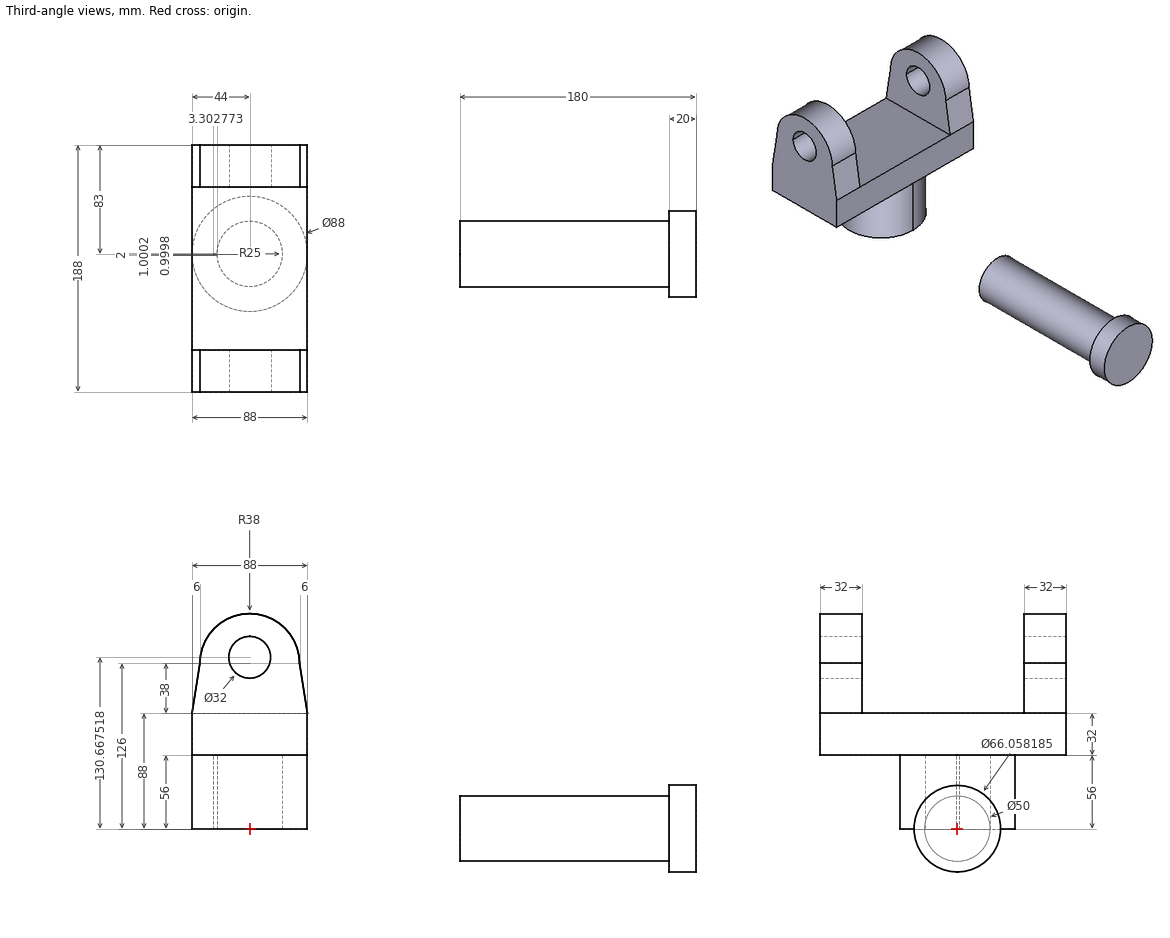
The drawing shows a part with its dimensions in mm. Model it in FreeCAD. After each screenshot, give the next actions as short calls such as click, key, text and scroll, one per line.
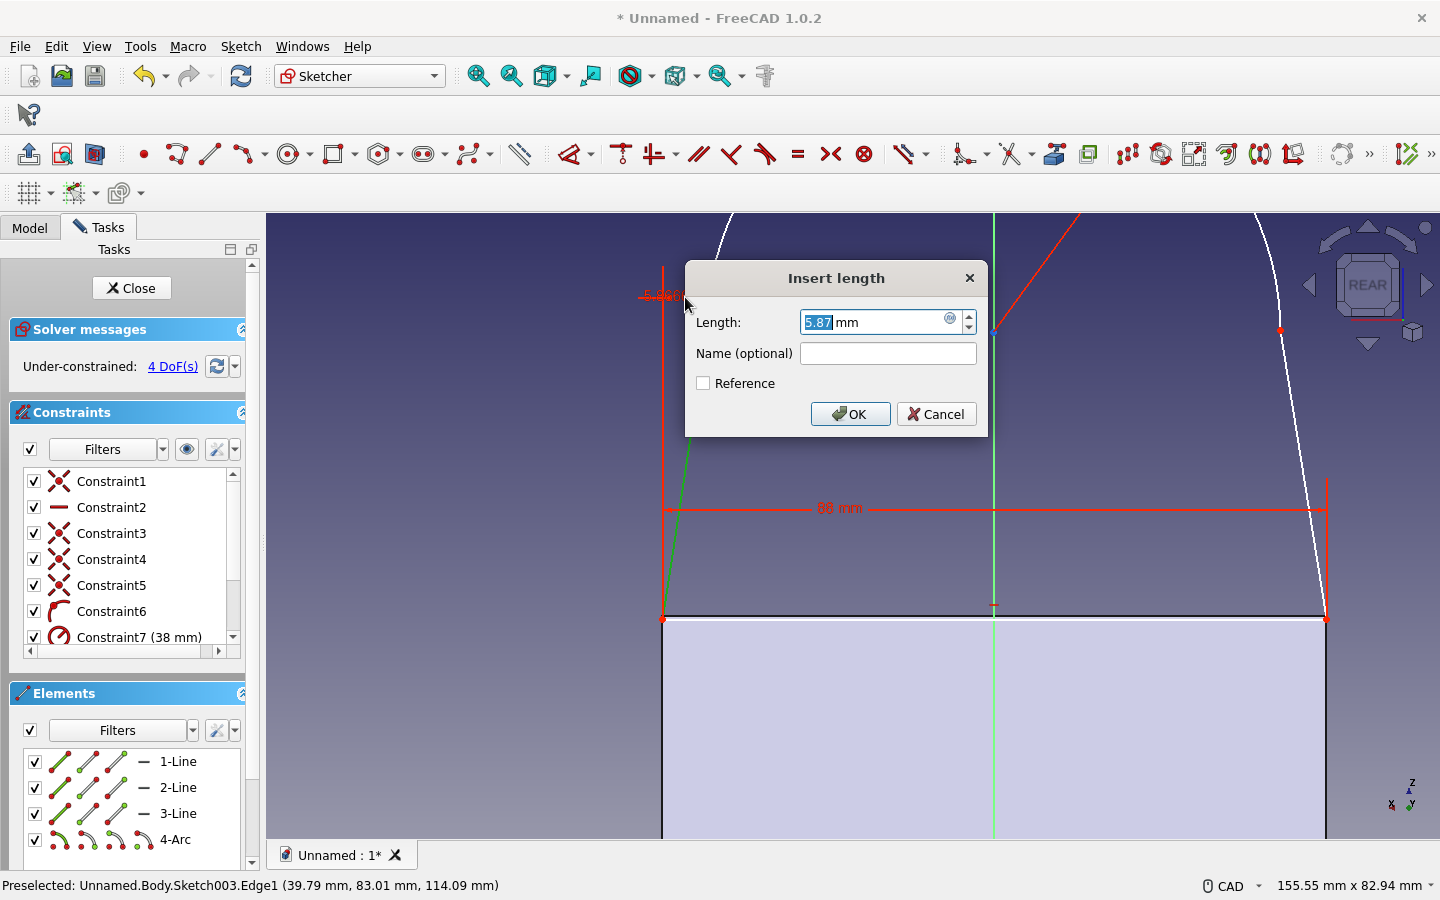
text(6)
key(Return)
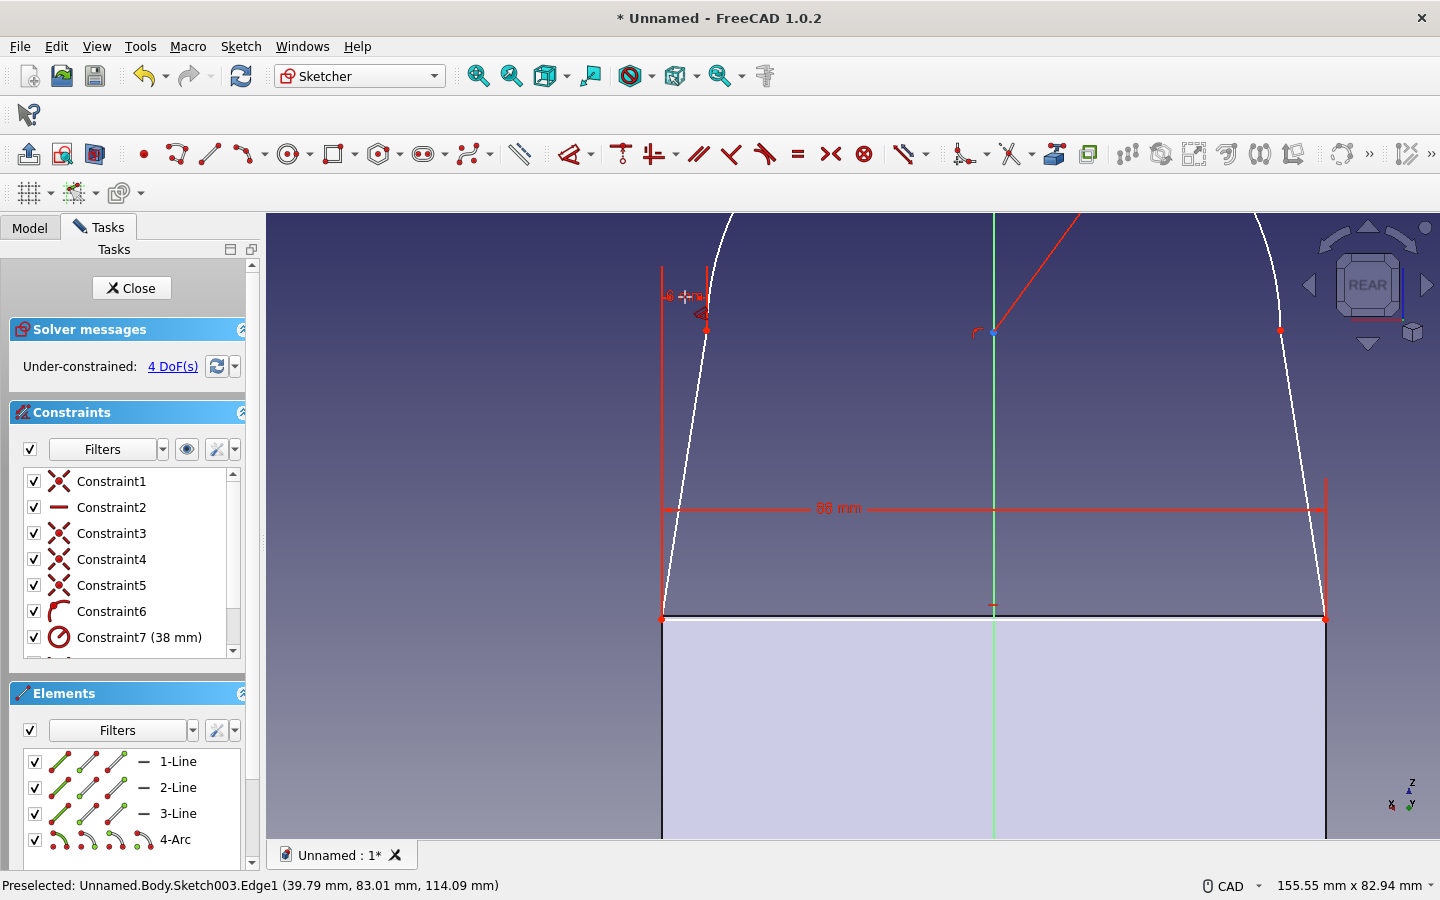
click(662, 620)
click(628, 715)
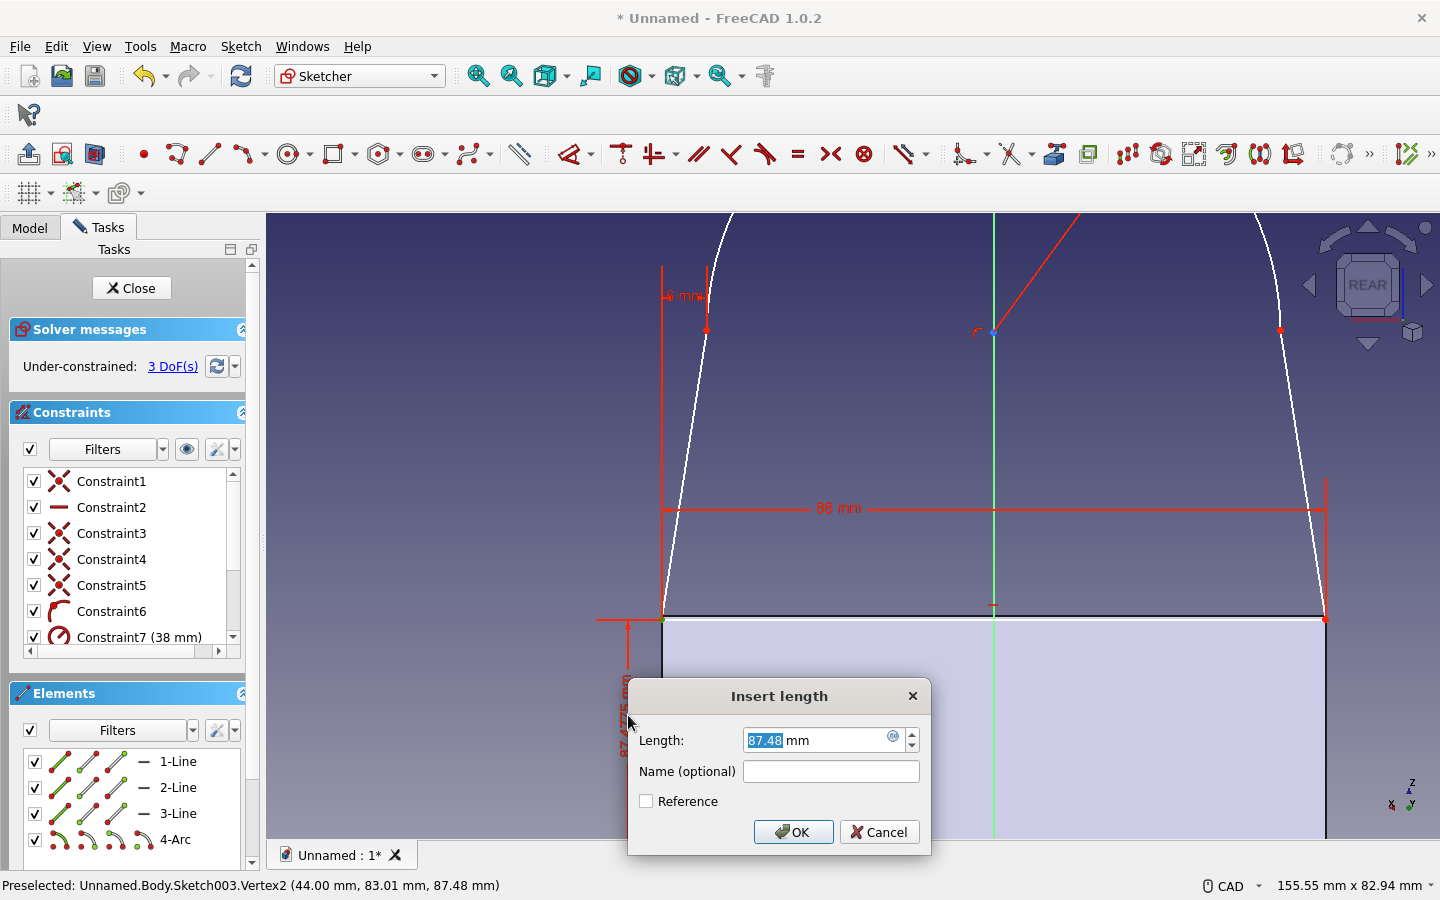
text(88)
key(Return)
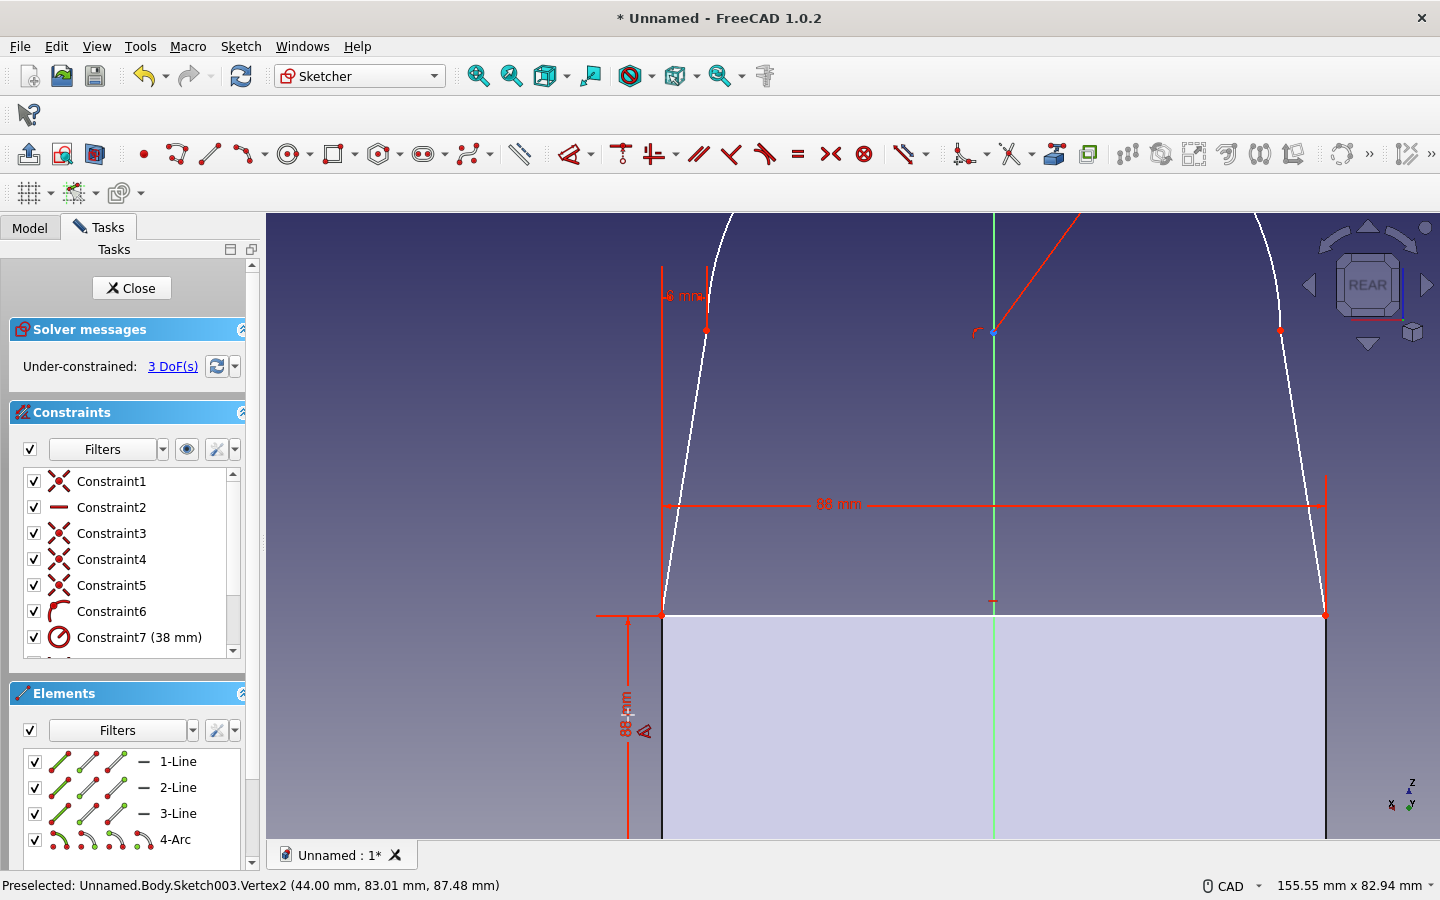
click(693, 416)
click(628, 473)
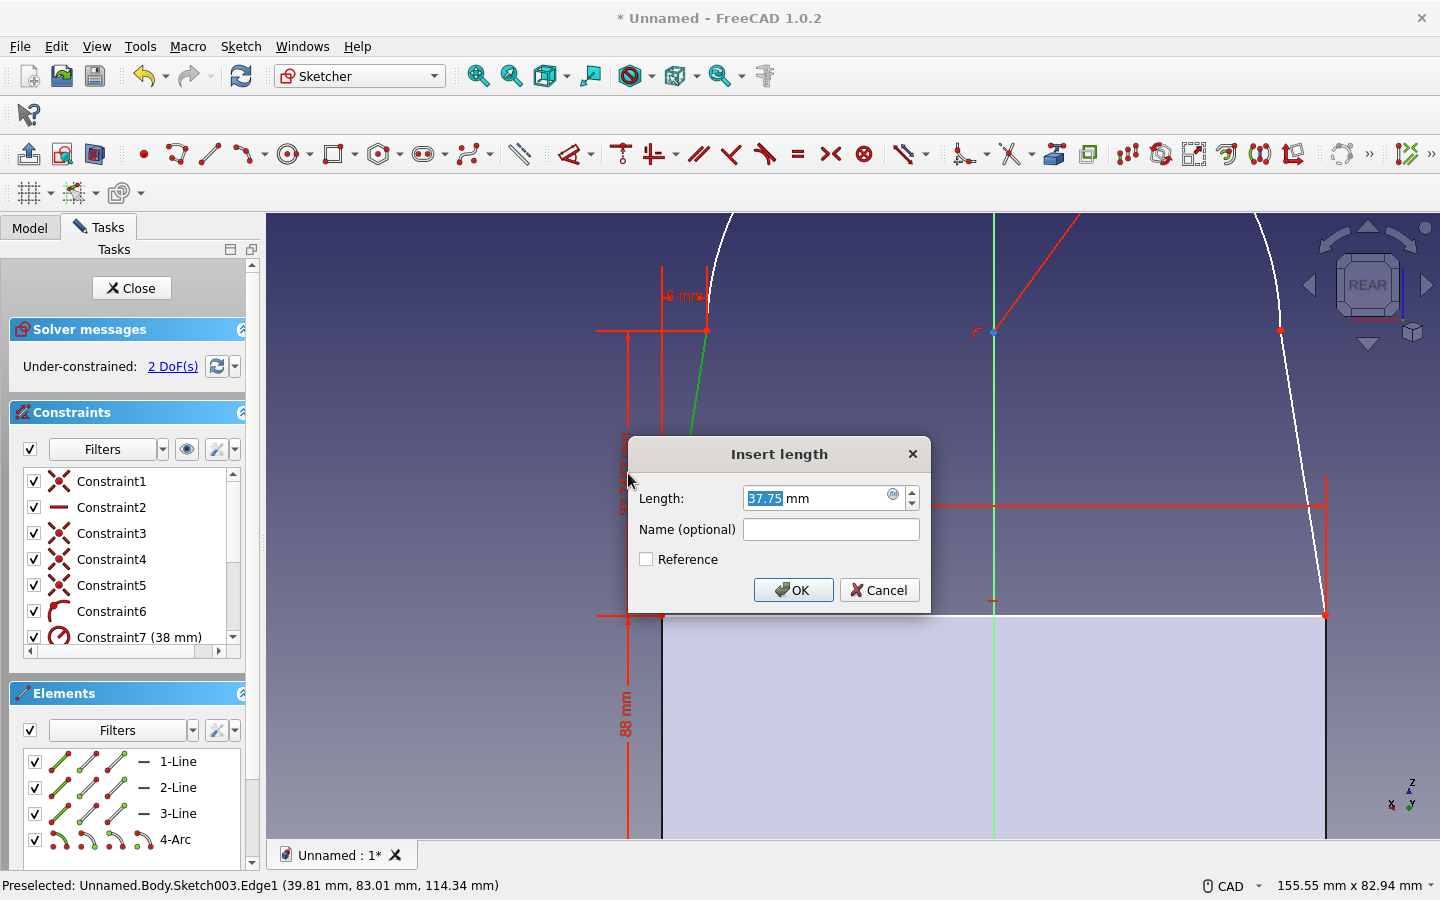
text(38)
key(Return)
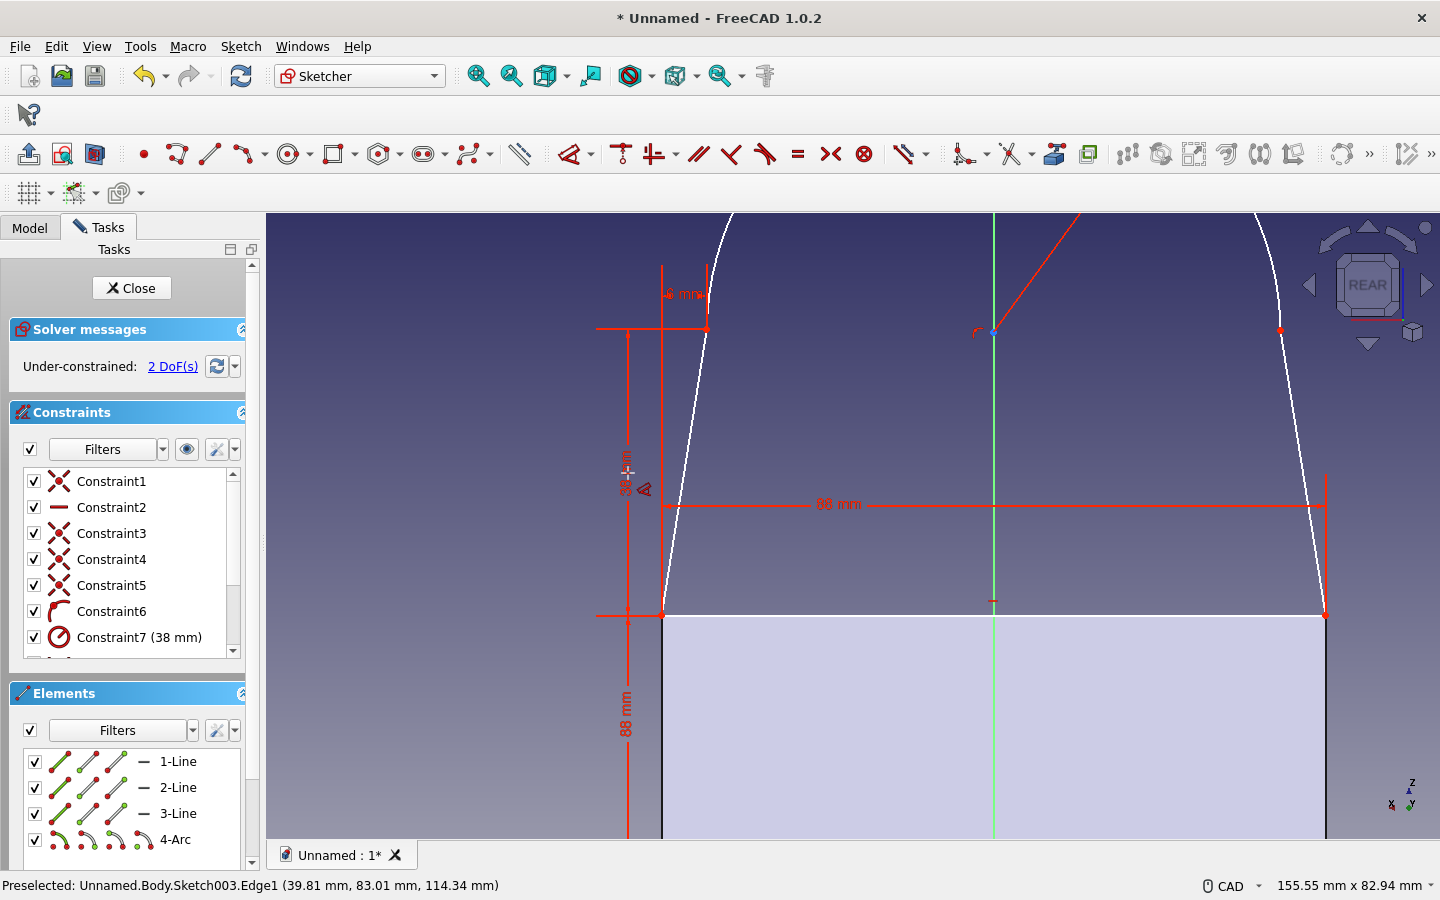
scroll(694, 468, down, 6)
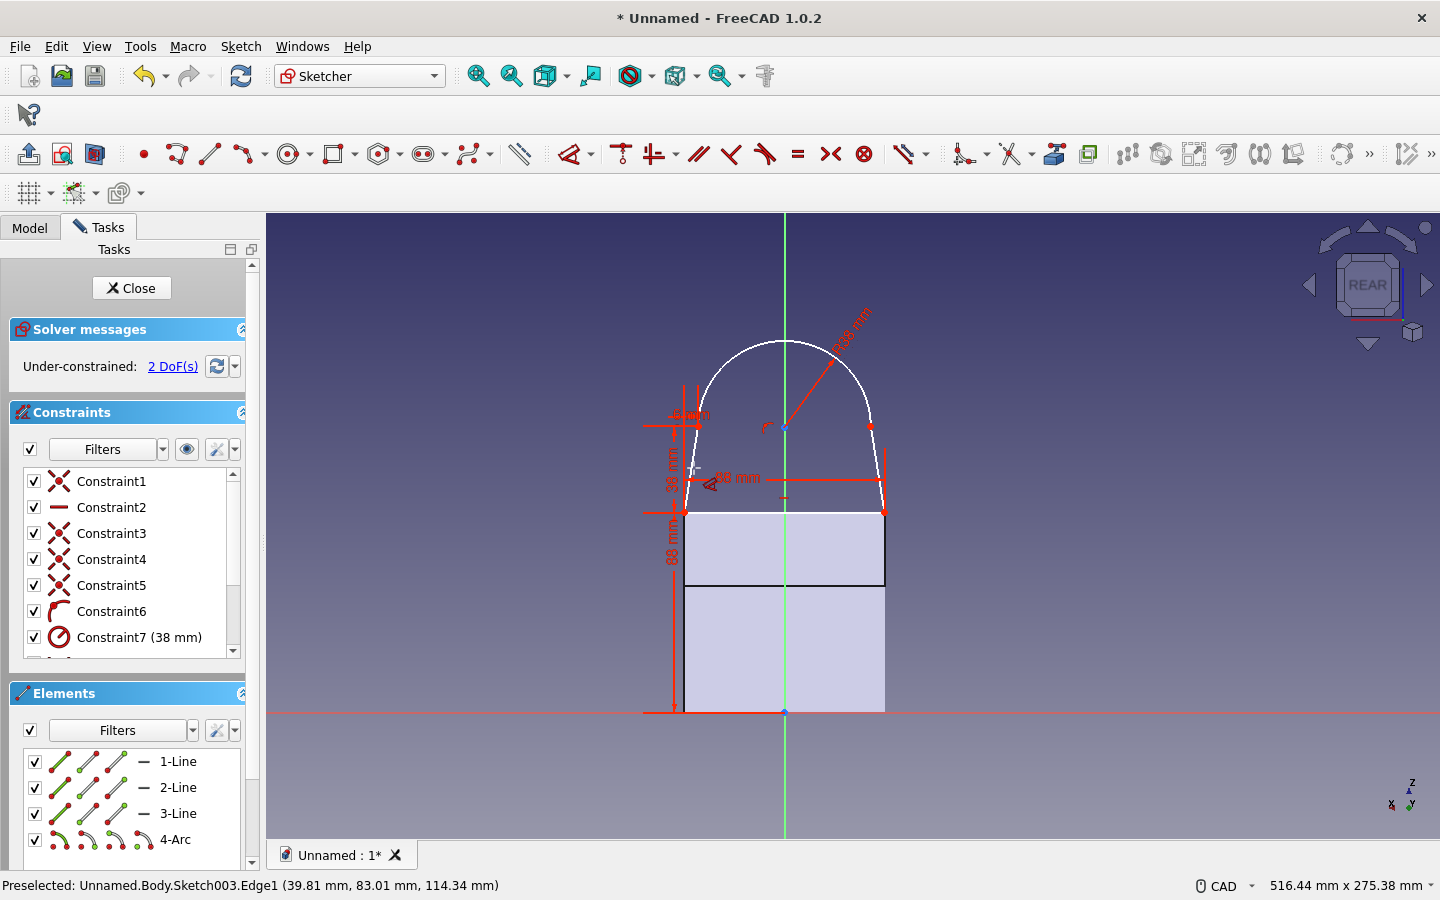
click(880, 487)
click(919, 470)